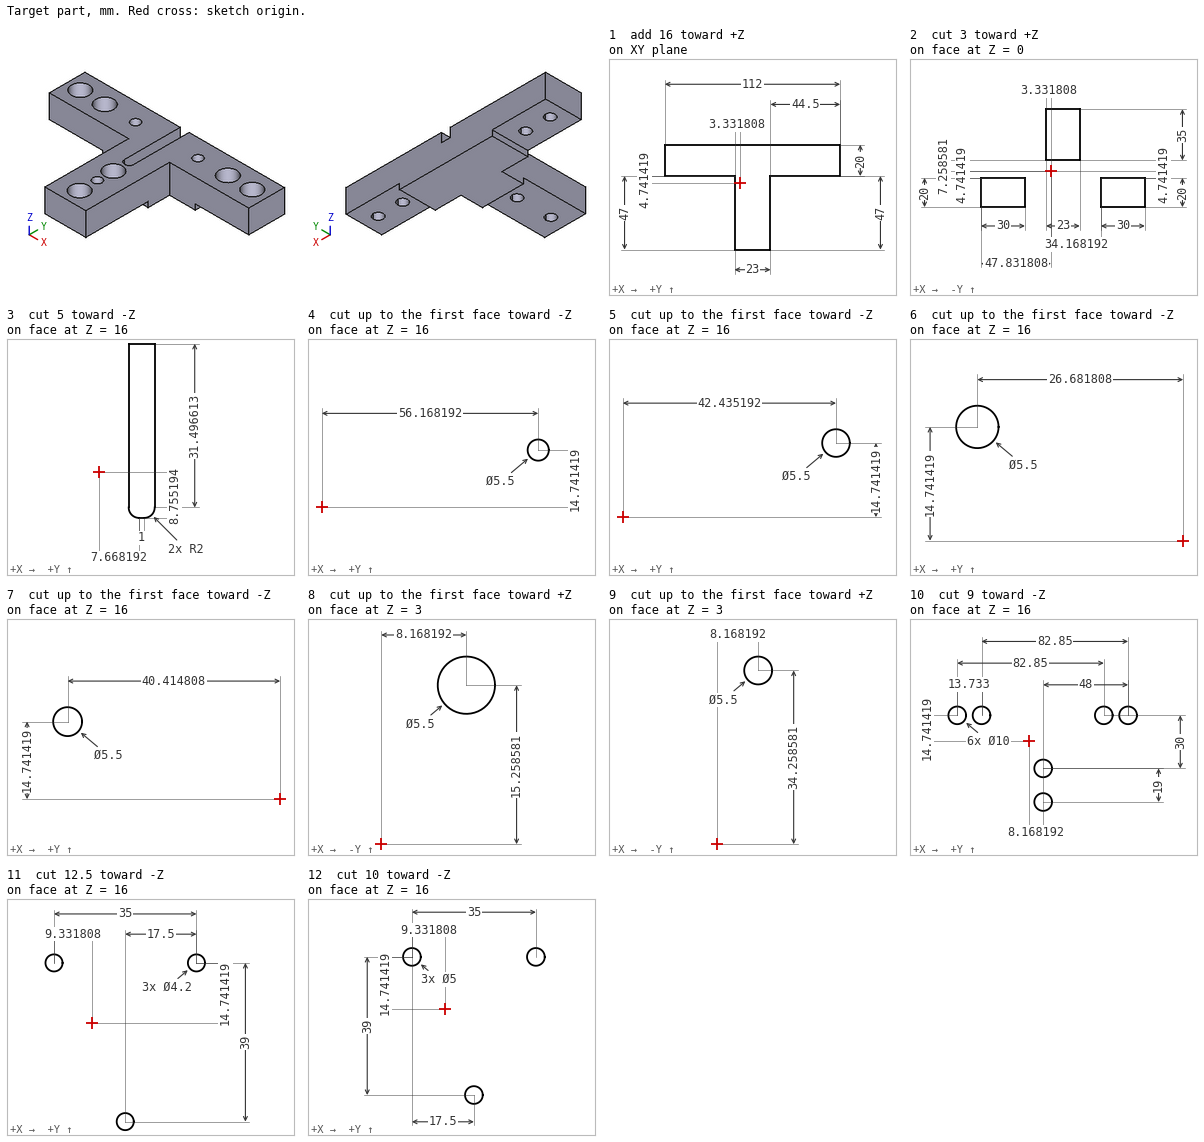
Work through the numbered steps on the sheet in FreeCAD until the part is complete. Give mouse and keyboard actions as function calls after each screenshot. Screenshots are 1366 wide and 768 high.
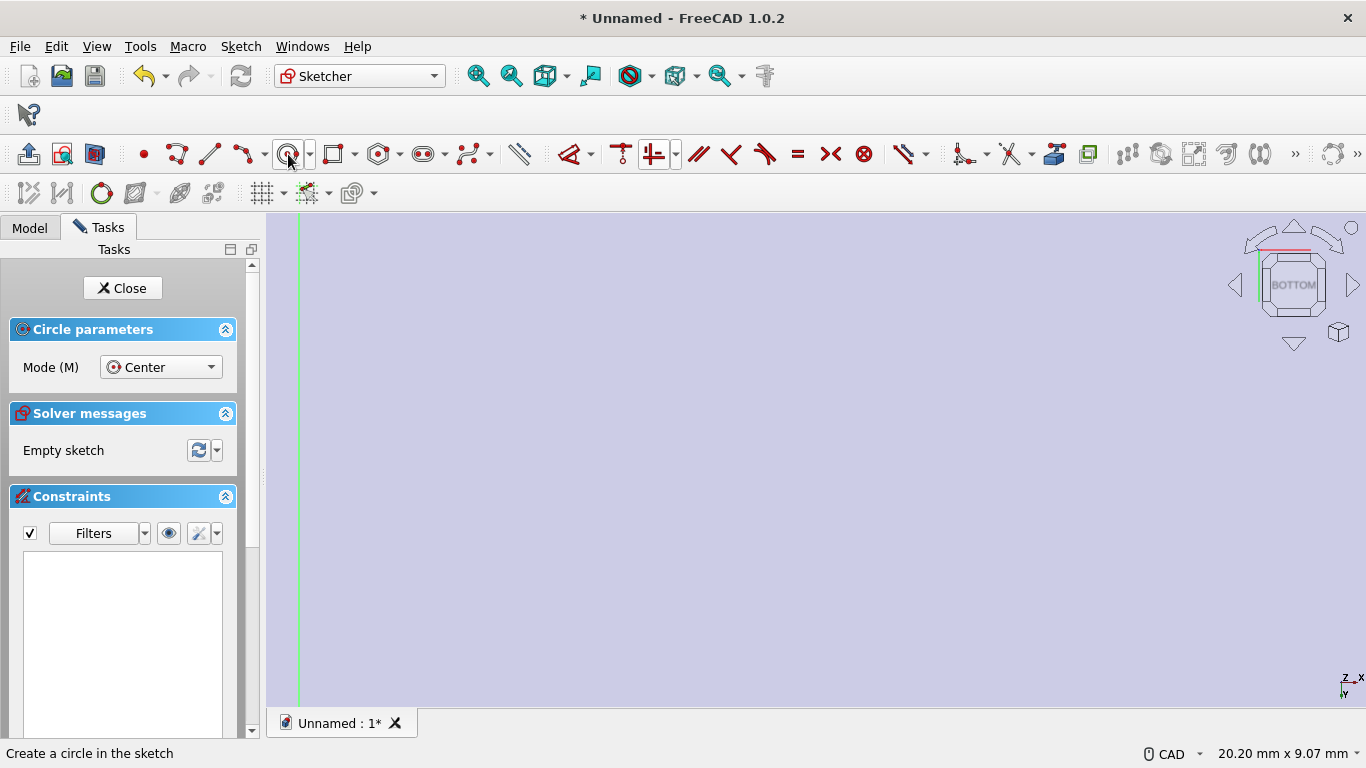
click(744, 458)
move(850, 352)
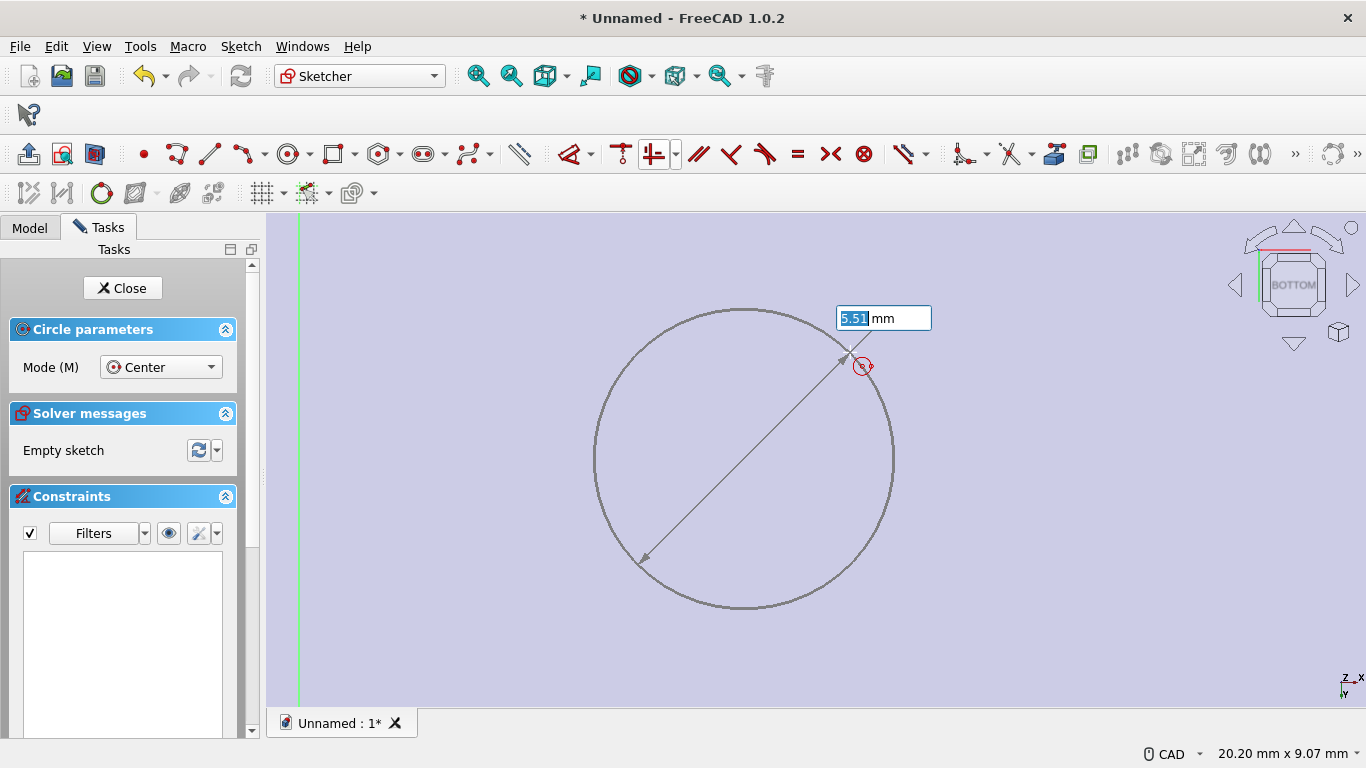
text(5.5)
key(Return)
key(Escape)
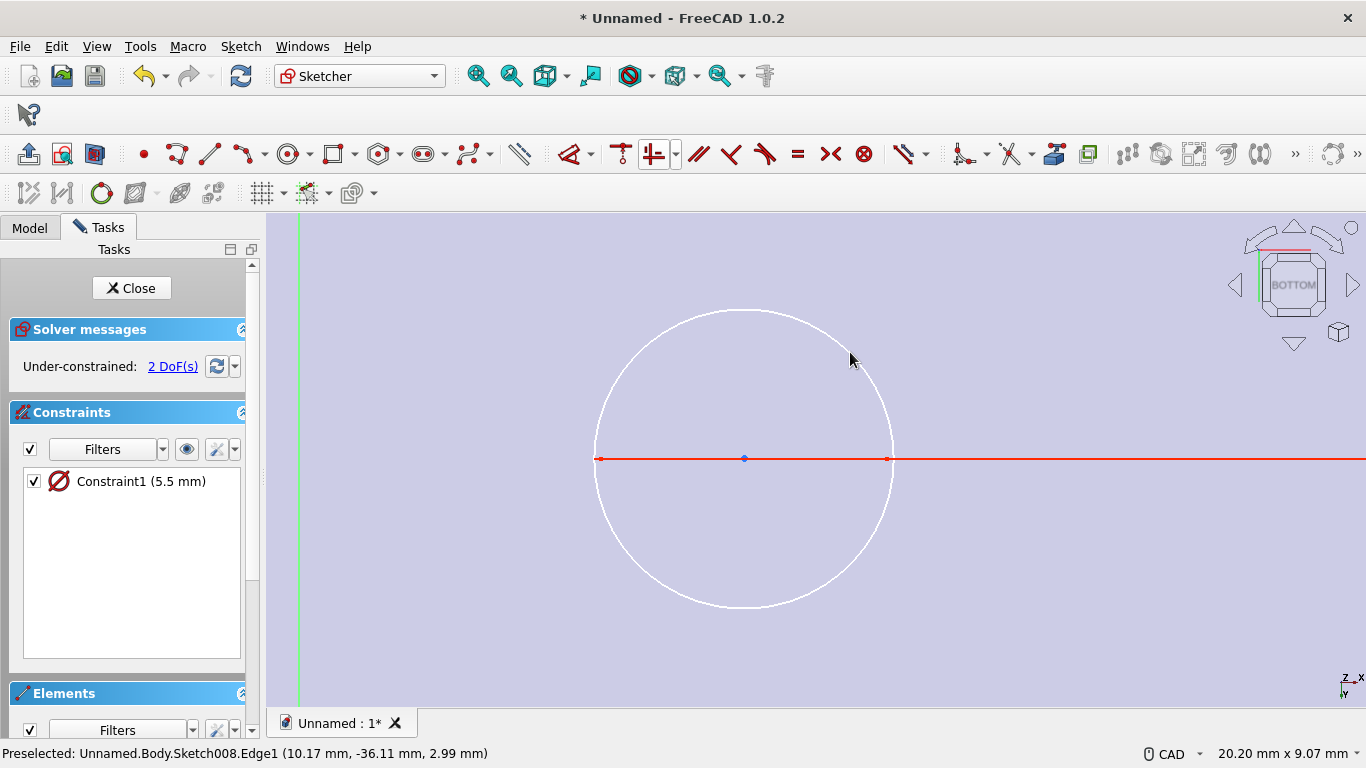
click(568, 154)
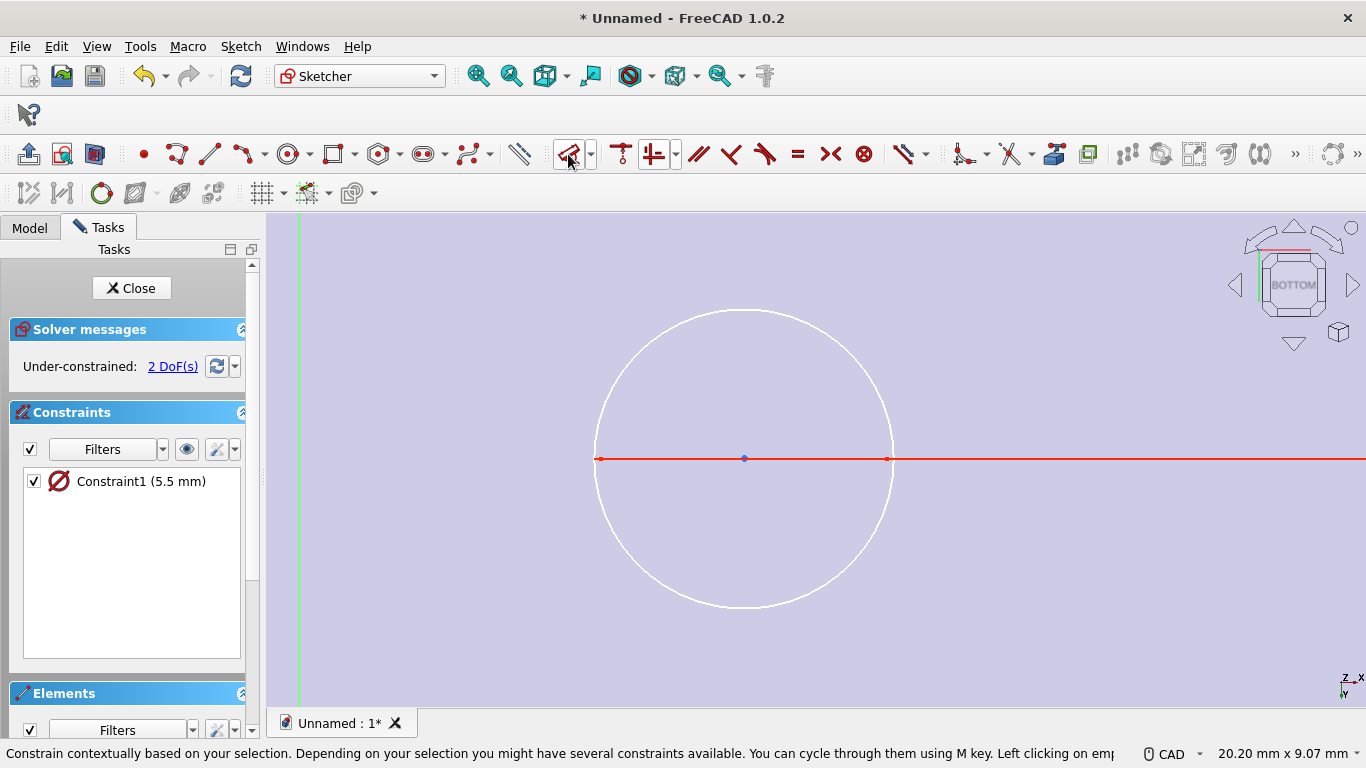
click(744, 459)
click(522, 425)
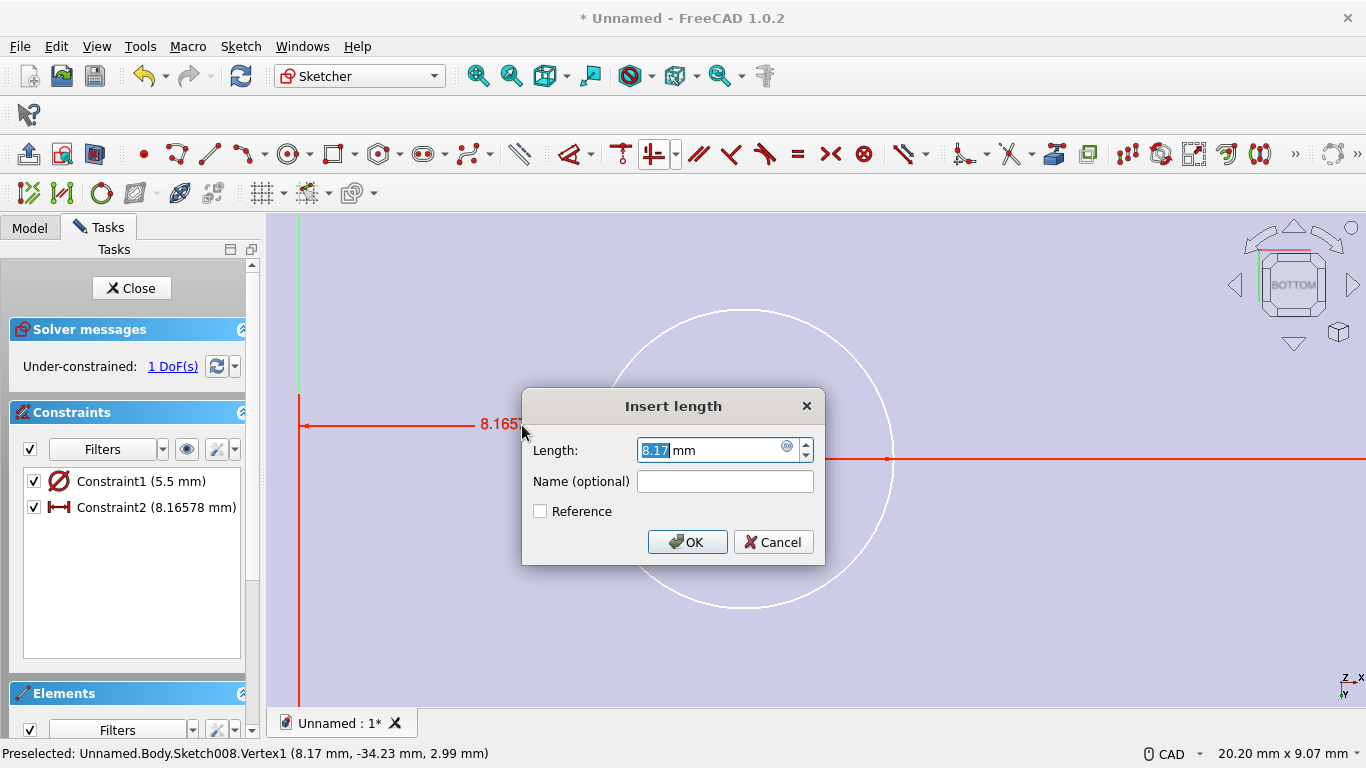
text(8.168192)
key(Return)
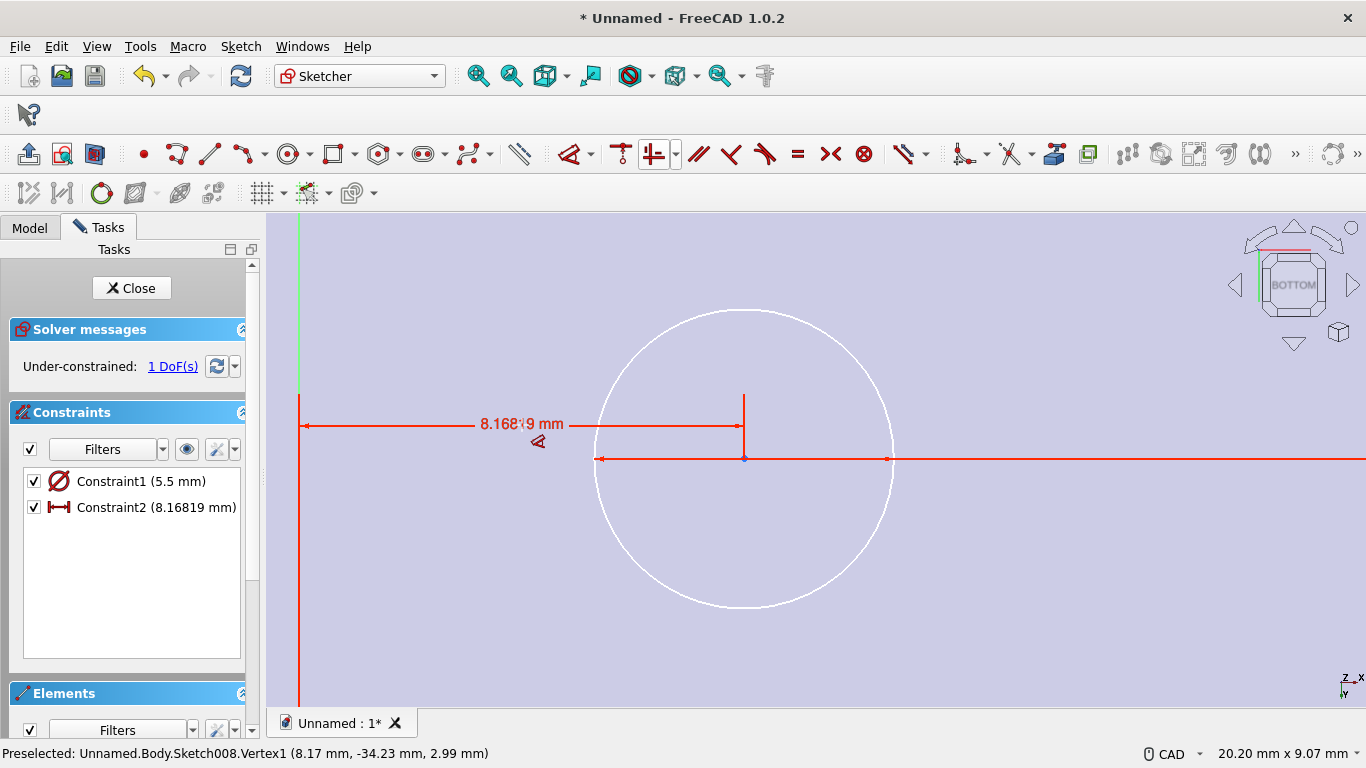
click(744, 459)
click(778, 569)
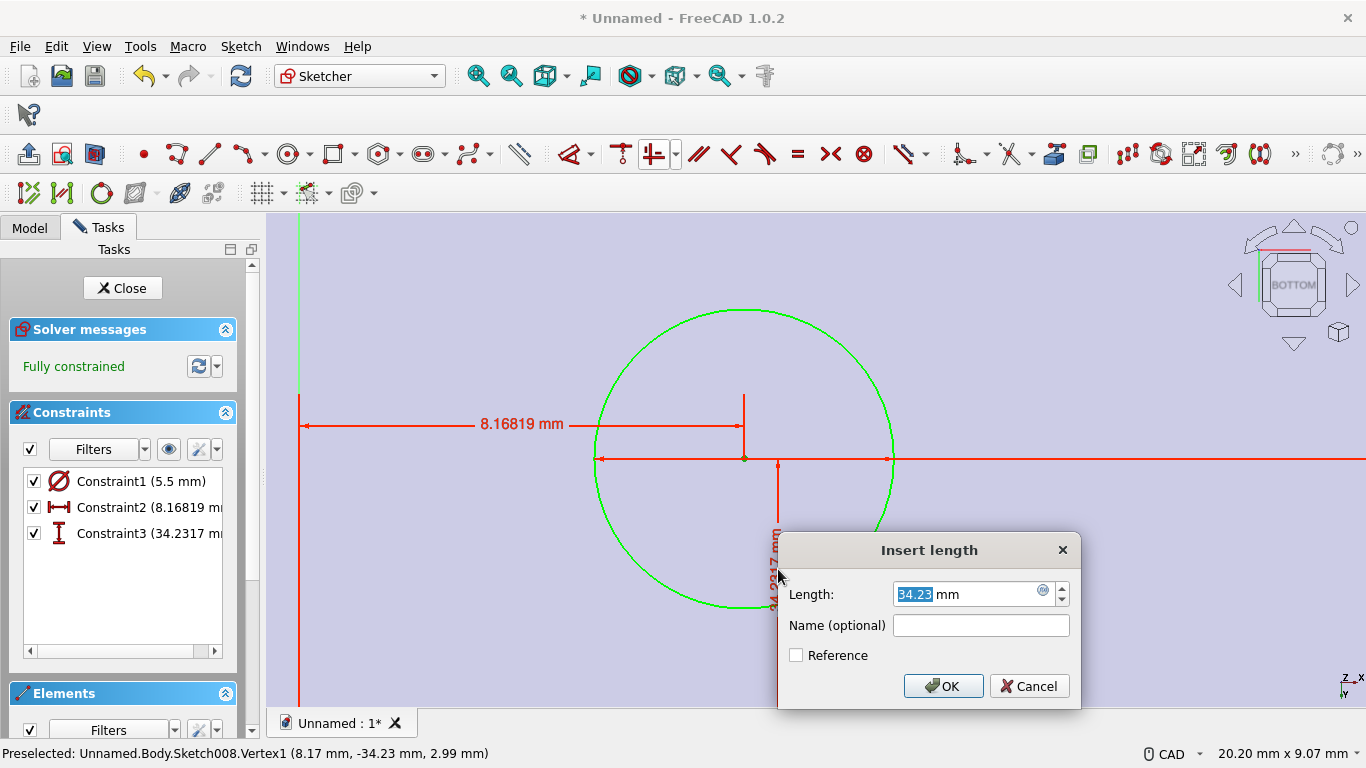
text(34.258581)
key(Return)
key(Escape)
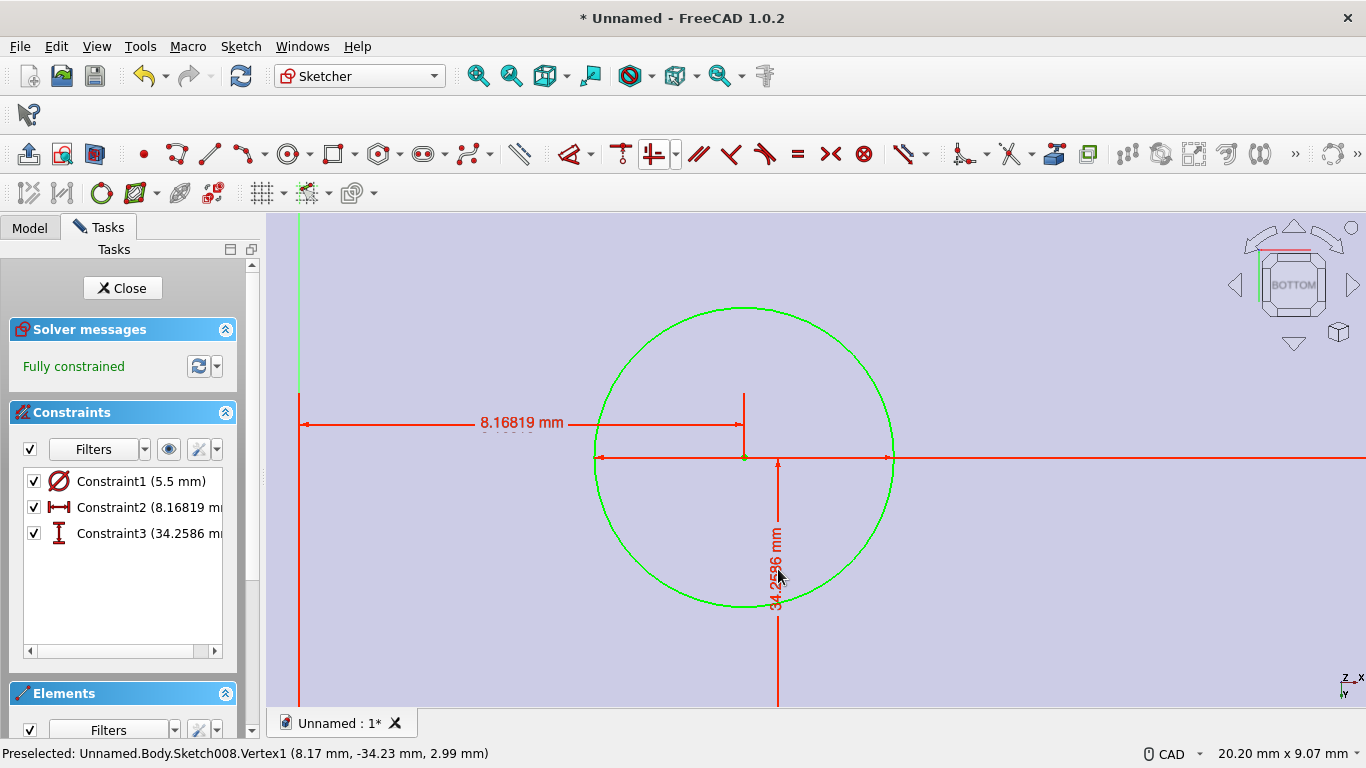
click(123, 288)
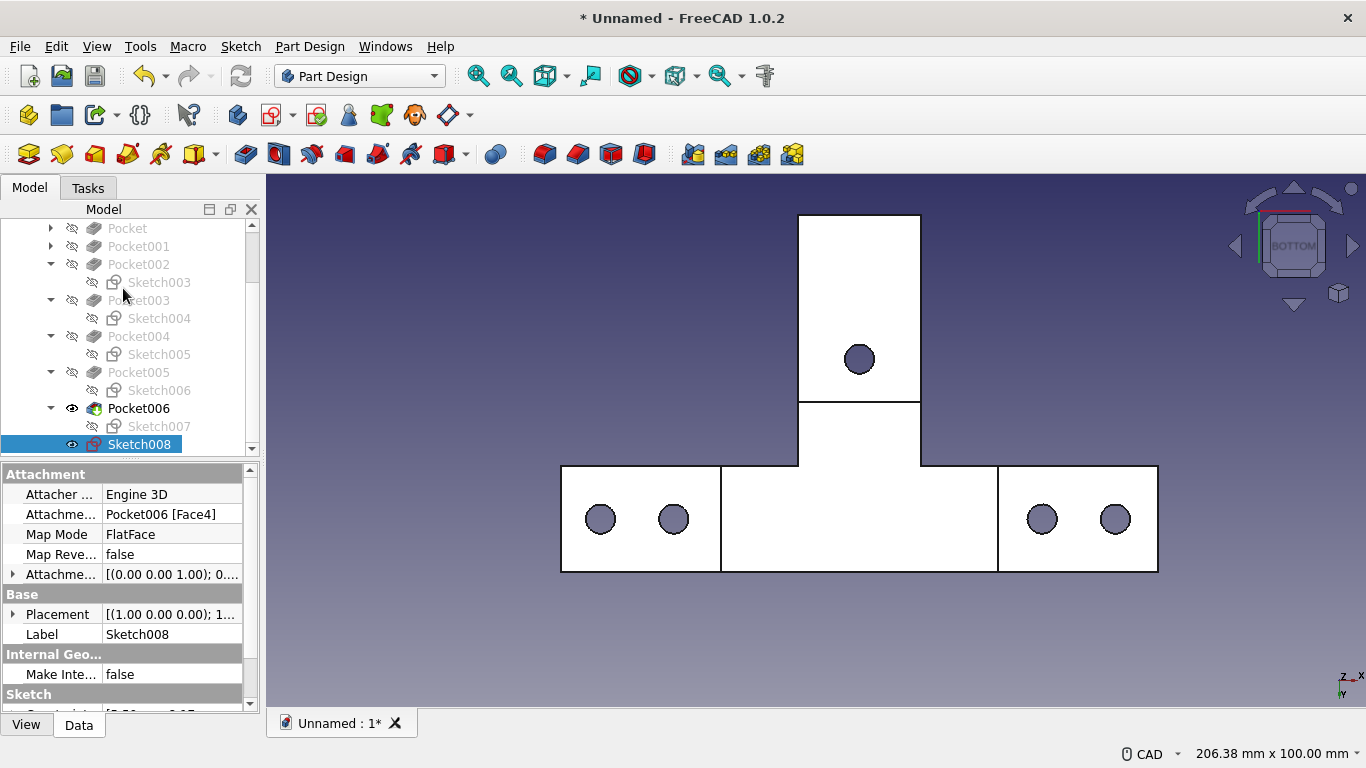
click(246, 154)